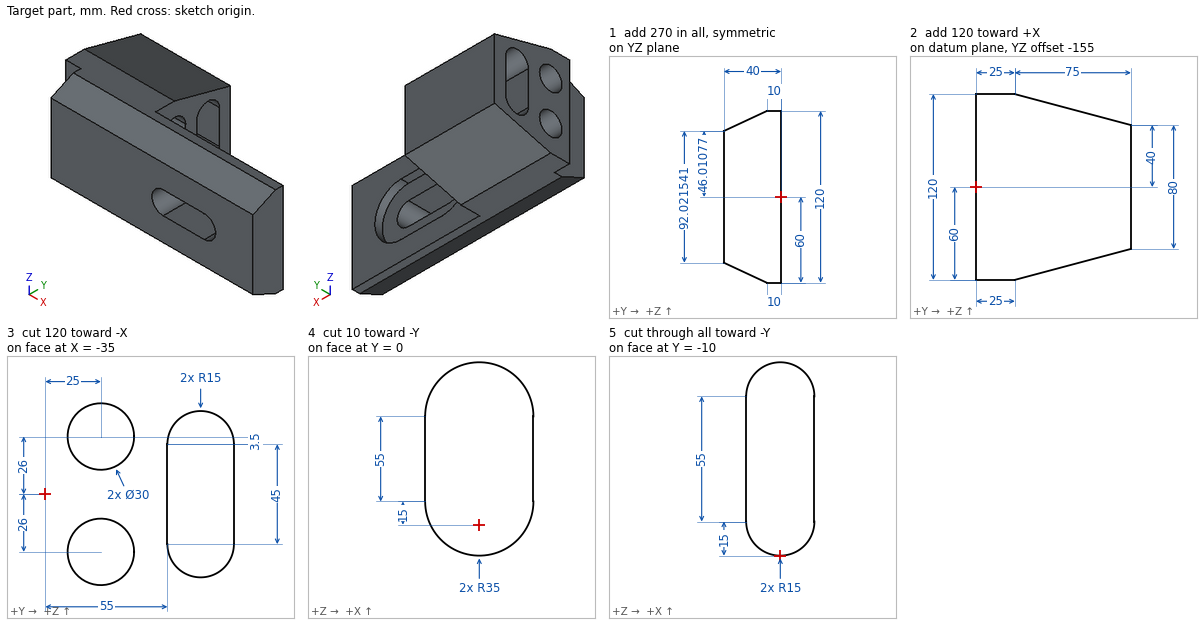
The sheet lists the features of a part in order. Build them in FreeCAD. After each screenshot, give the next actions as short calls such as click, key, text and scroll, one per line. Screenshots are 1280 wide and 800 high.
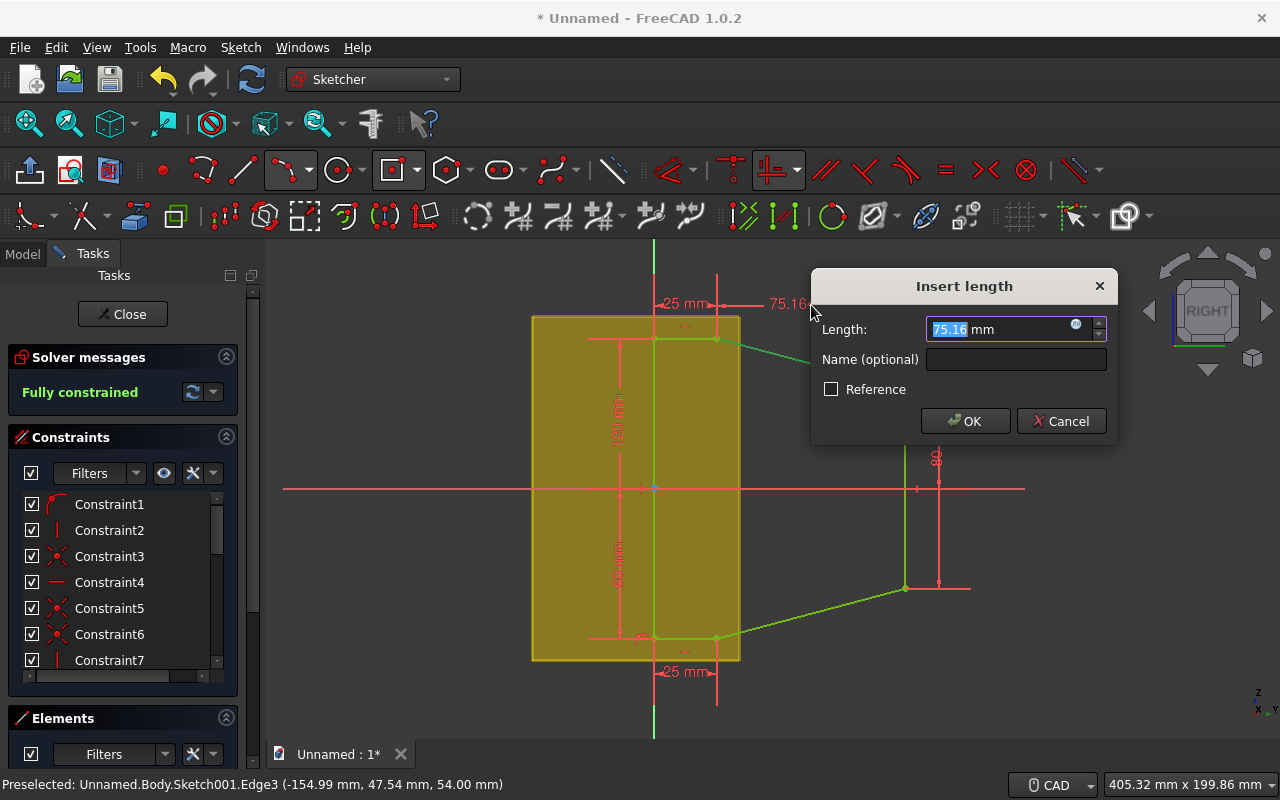
text(75)
key(Return)
key(Escape)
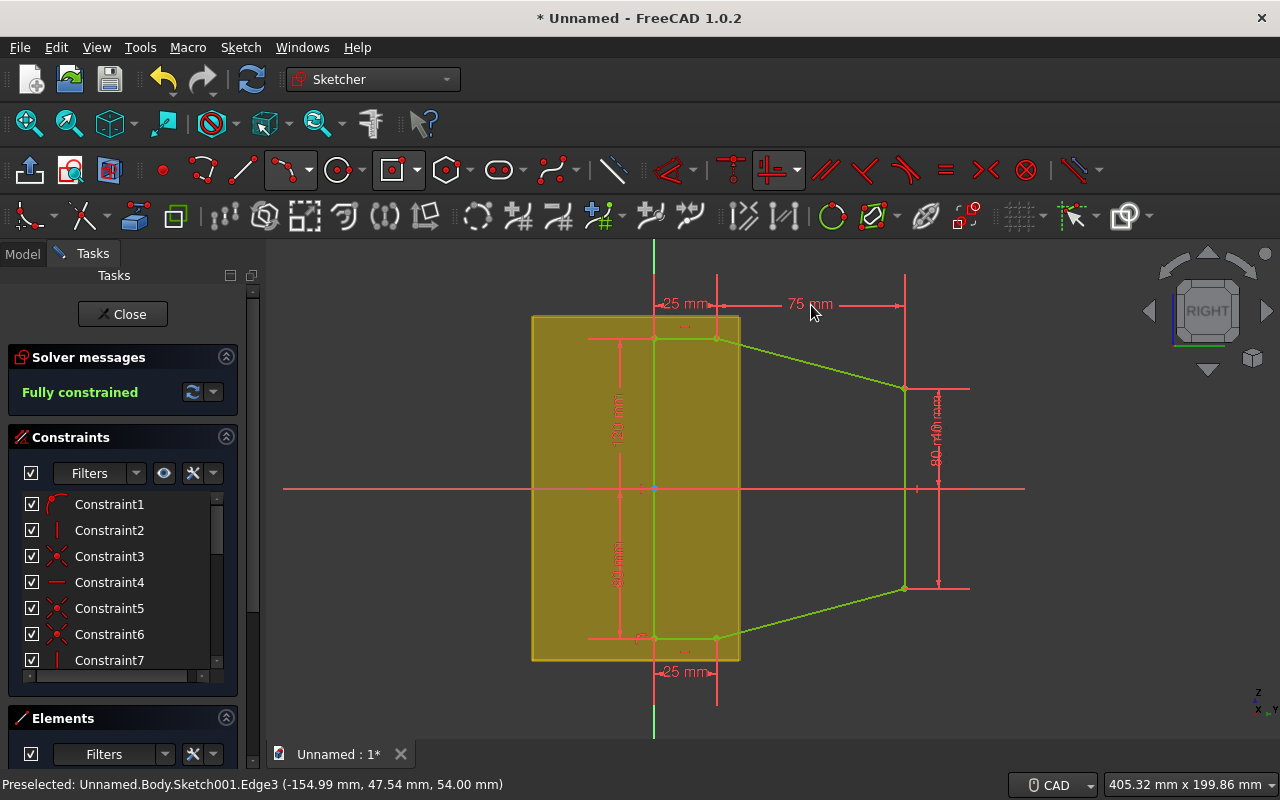
click(123, 314)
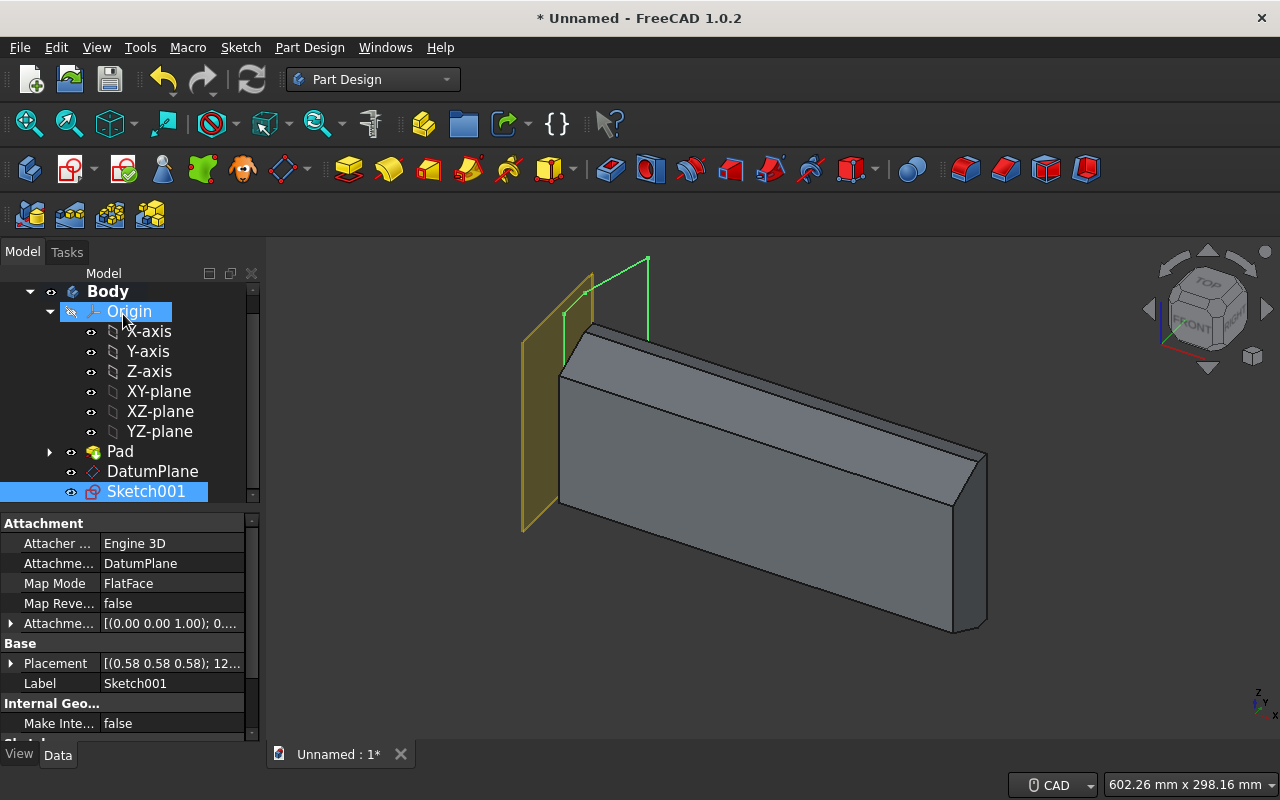
click(350, 170)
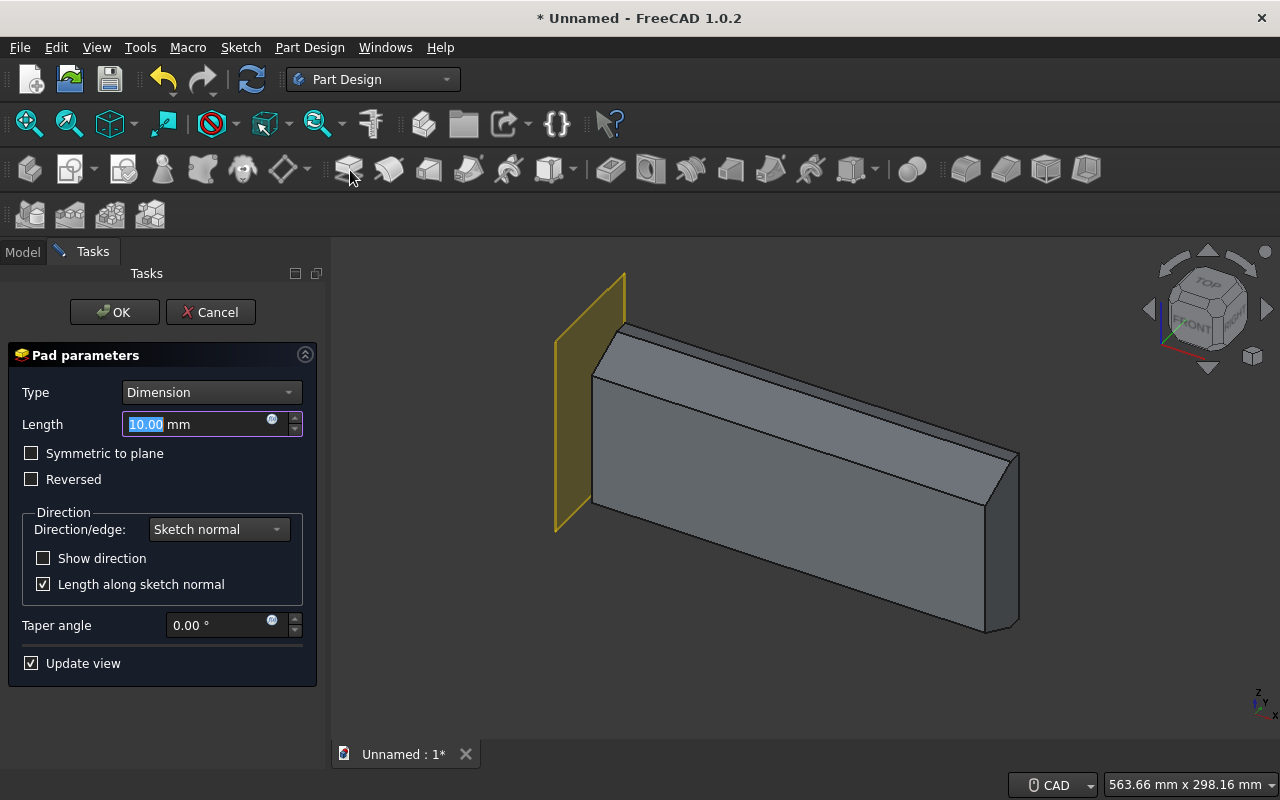
text(120)
key(Tab)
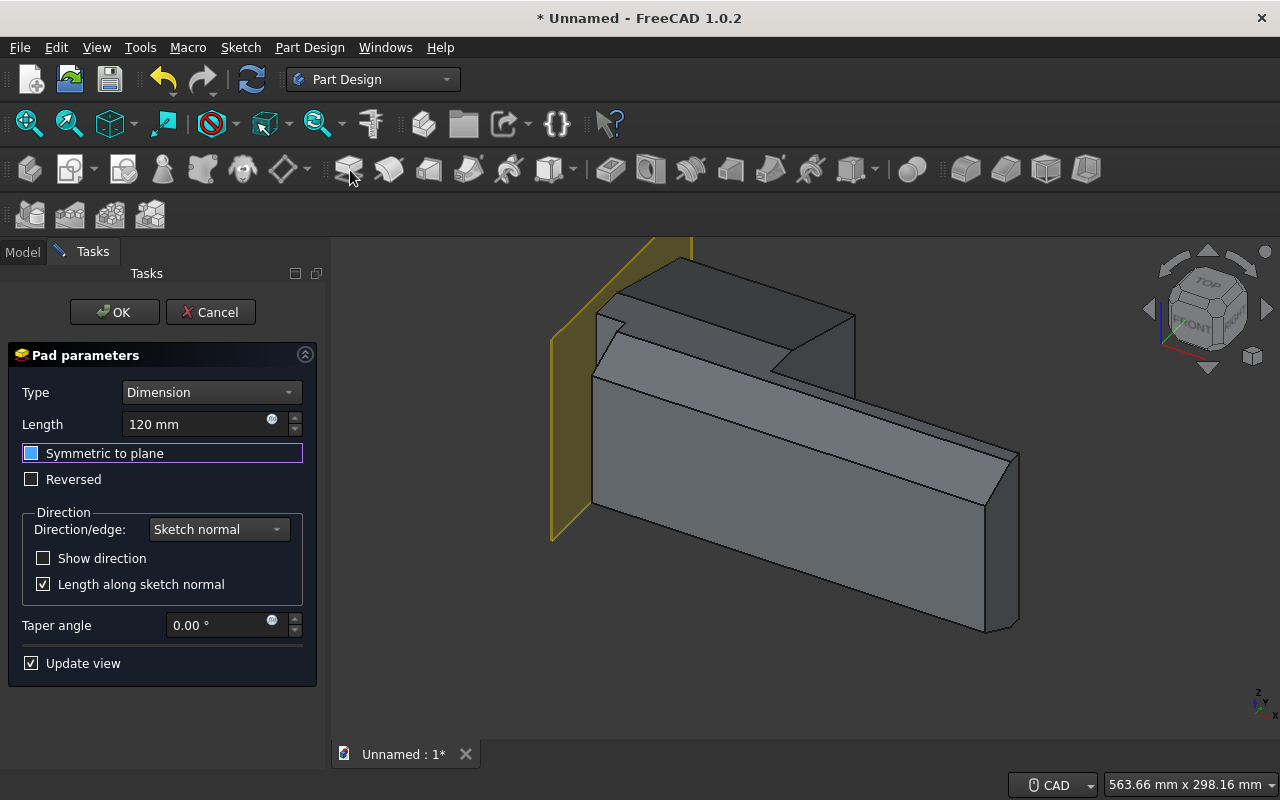
click(115, 312)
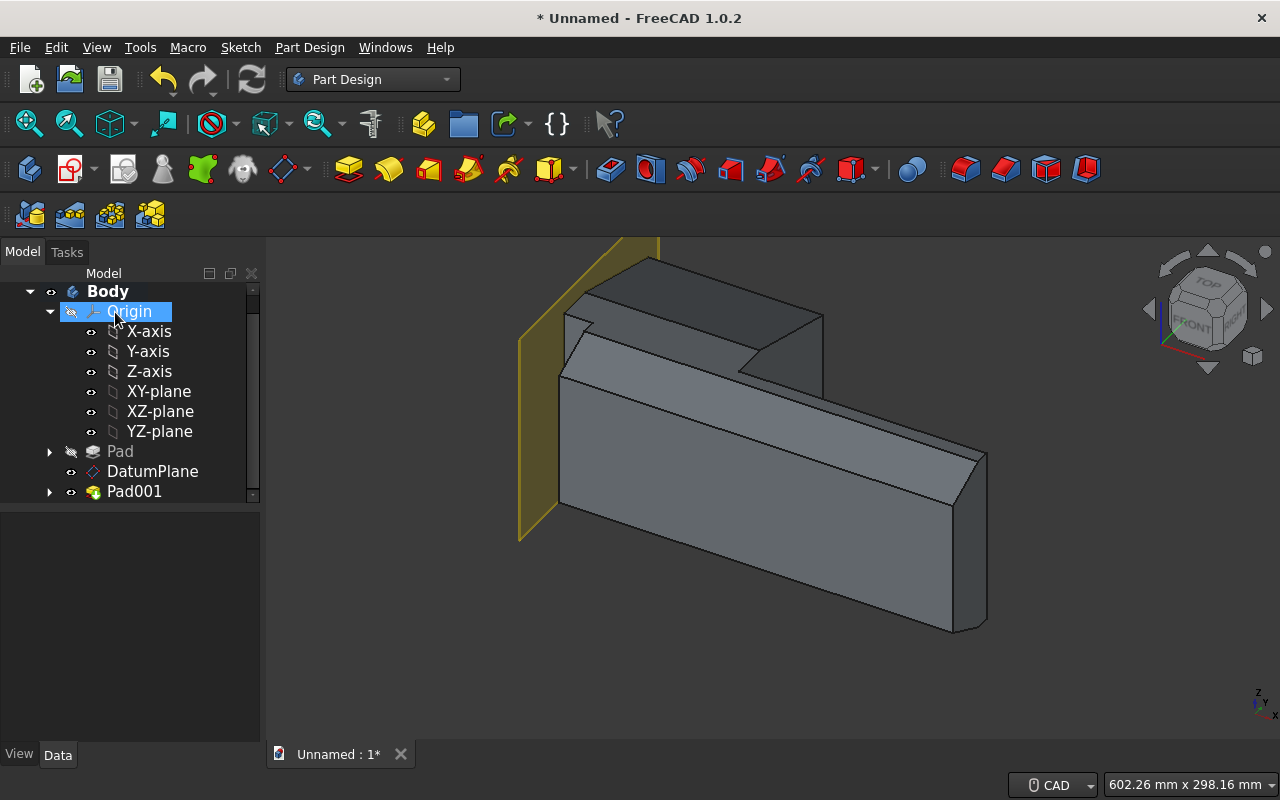
click(116, 472)
key(space)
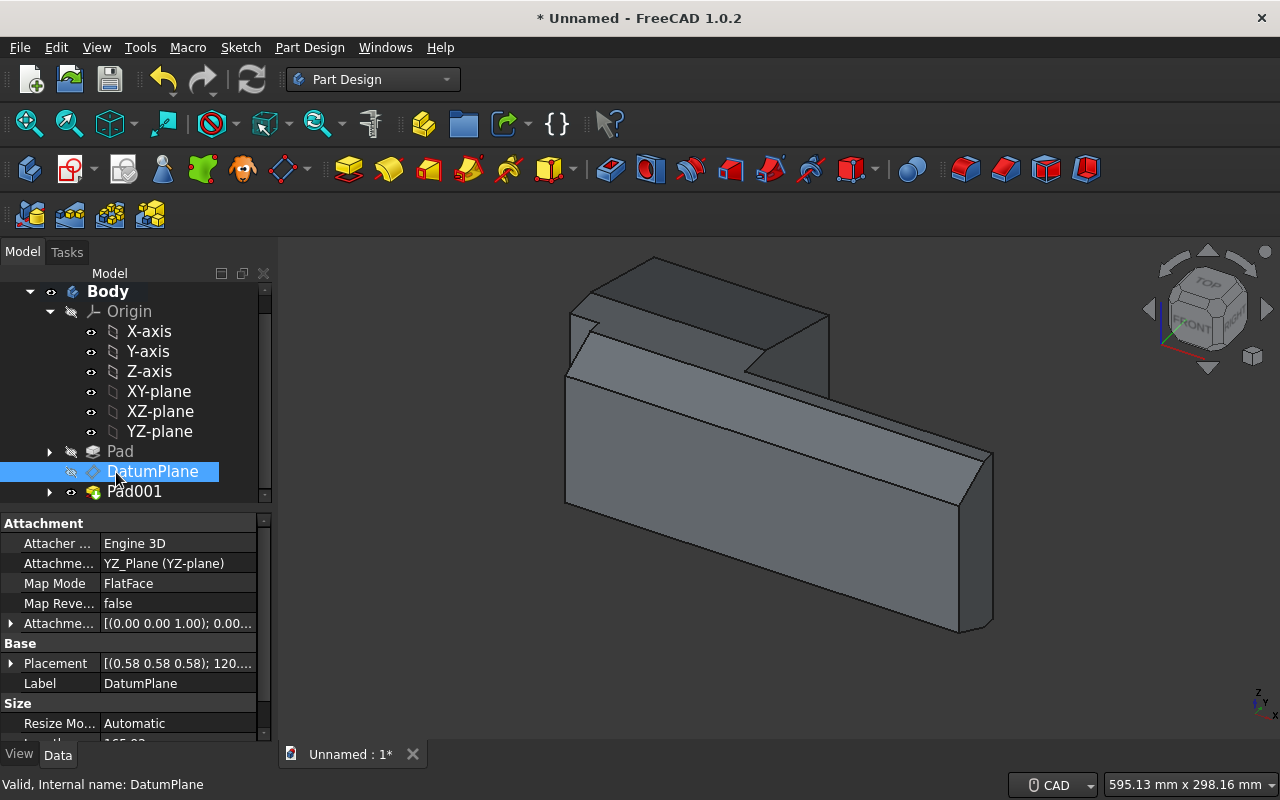
click(30, 124)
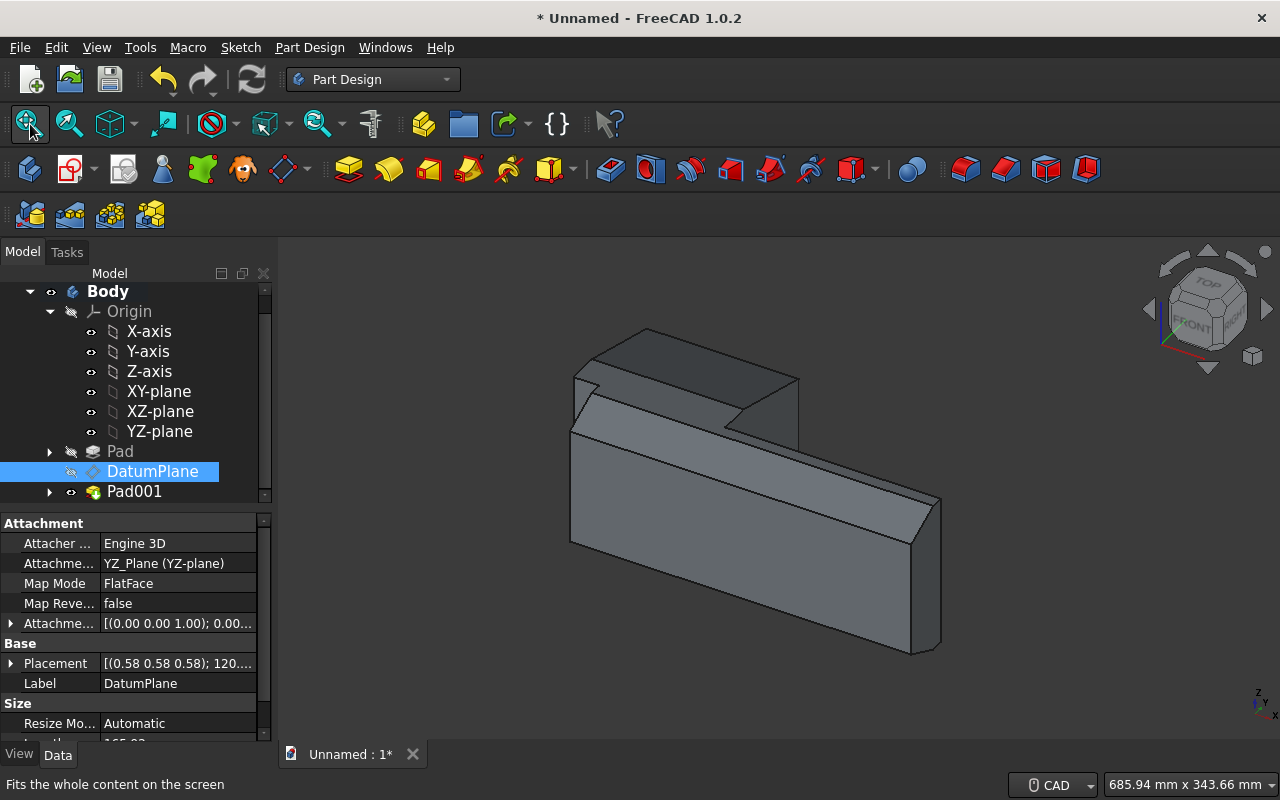
key(0)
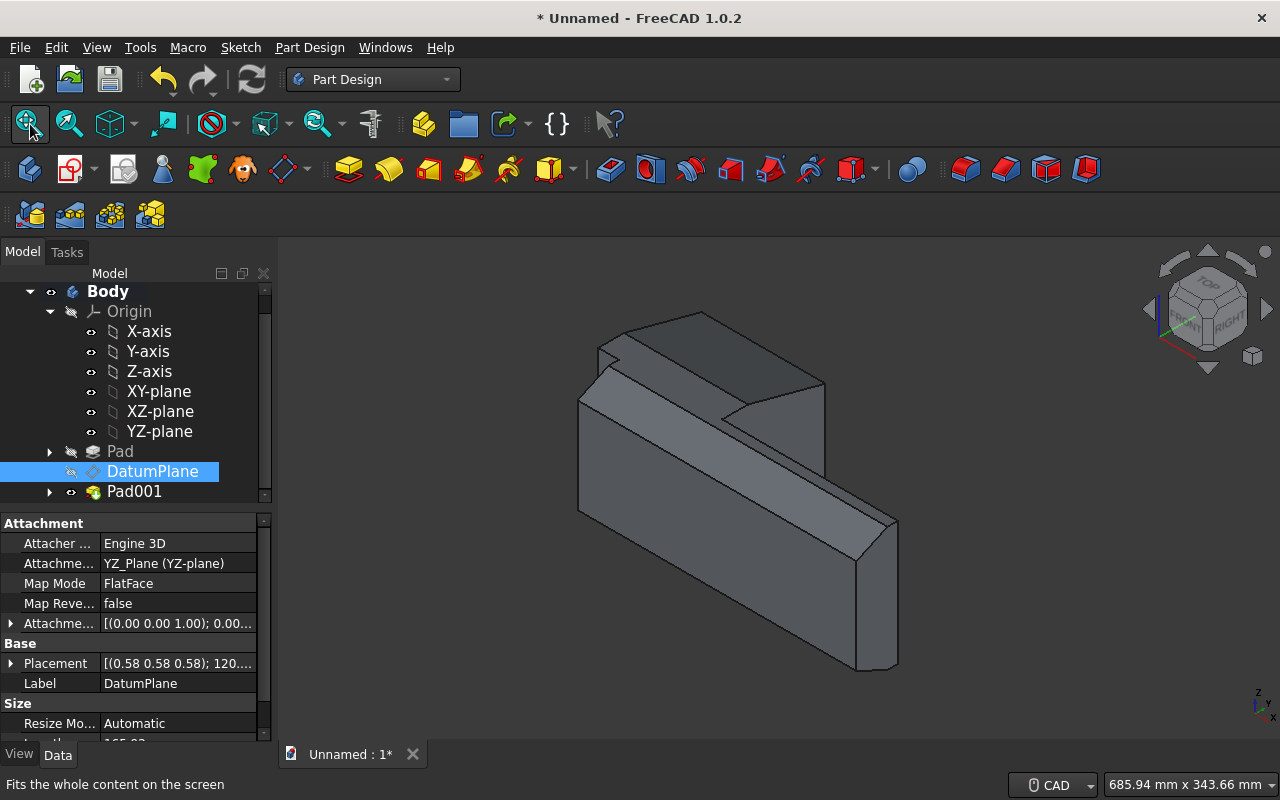
key(3)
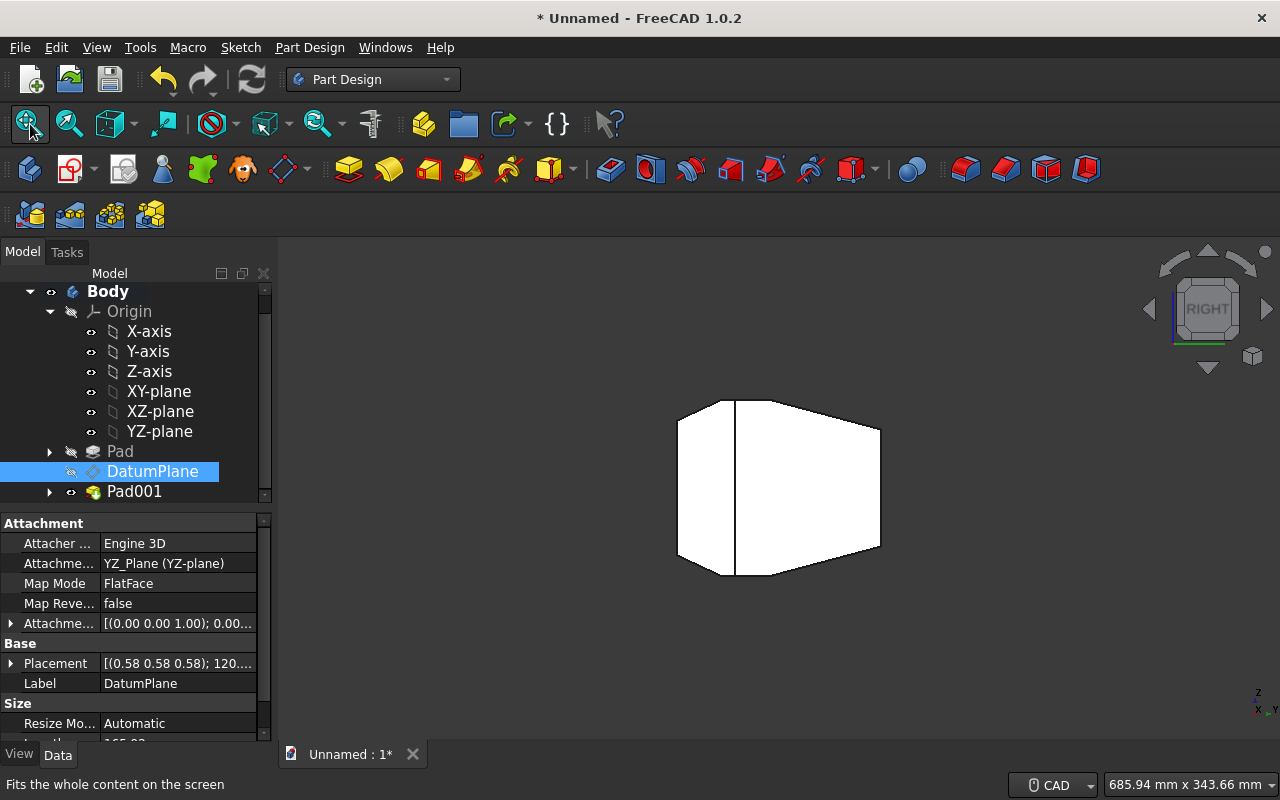
click(30, 124)